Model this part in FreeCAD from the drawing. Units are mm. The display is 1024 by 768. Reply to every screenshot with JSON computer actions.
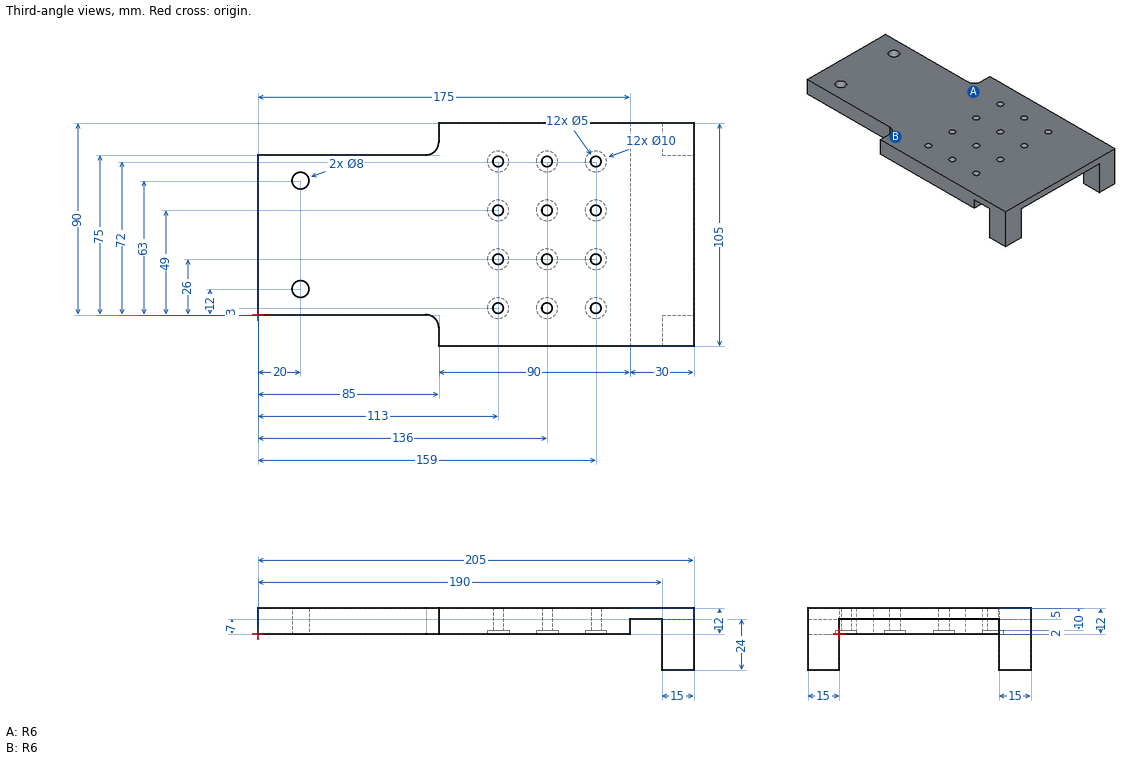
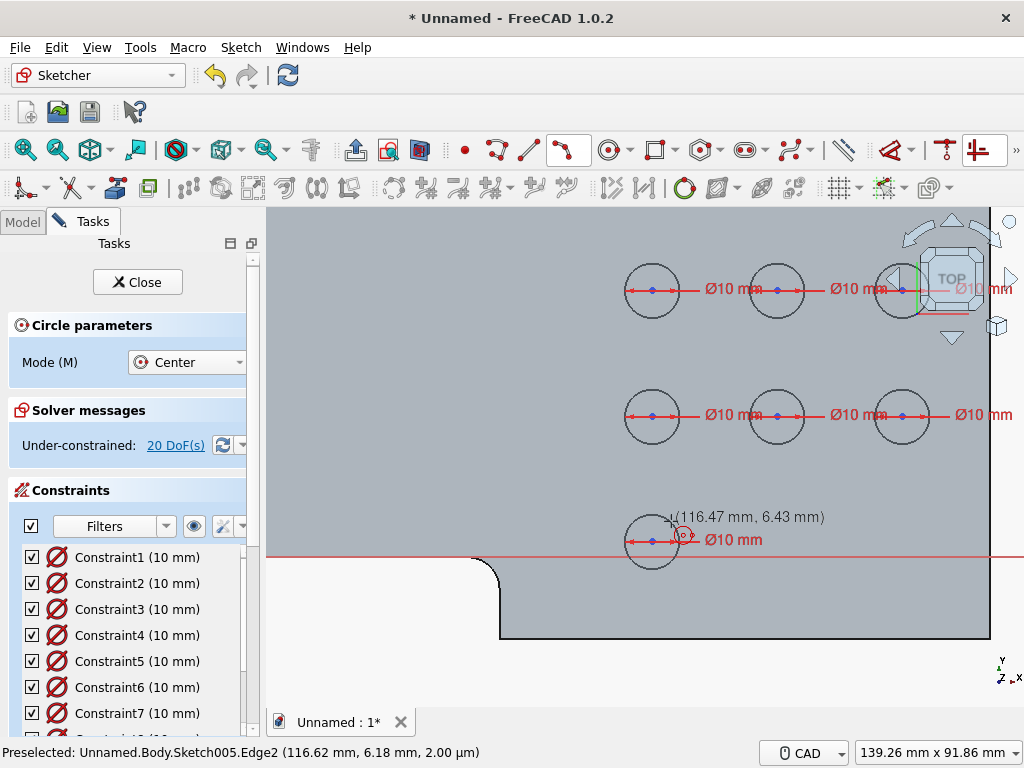
{"action": "left_click", "coordinate": [777, 541]}
{"action": "mouse_move", "coordinate": [797, 521]}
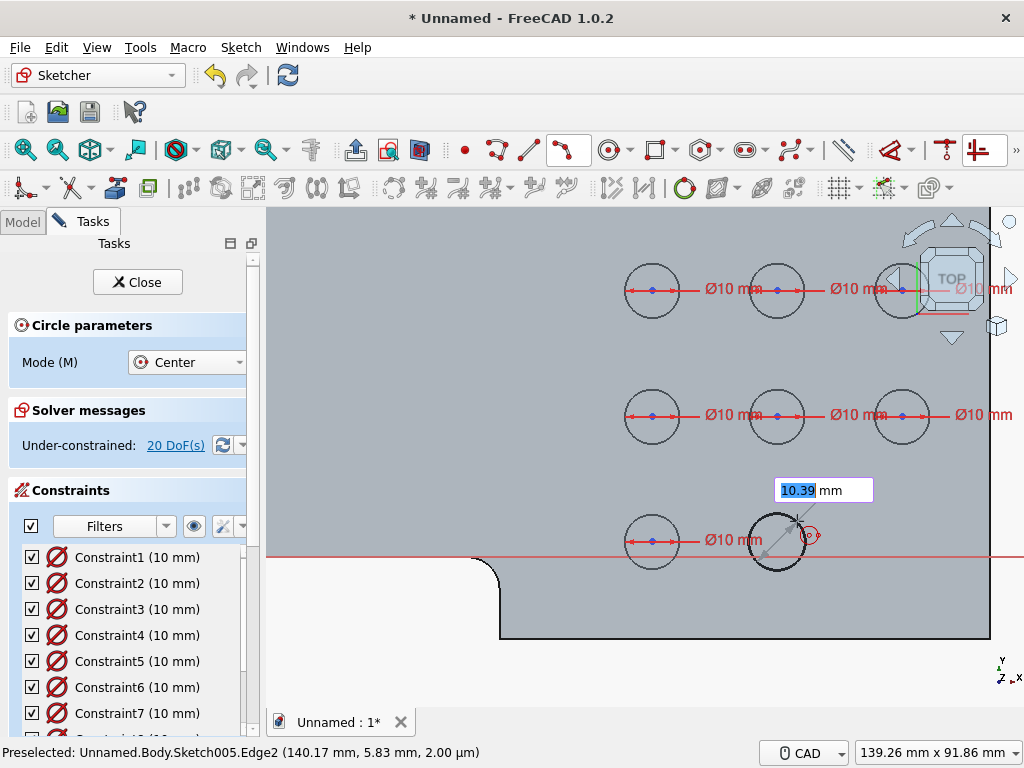
{"action": "type", "text": "10"}
{"action": "key", "text": "Return"}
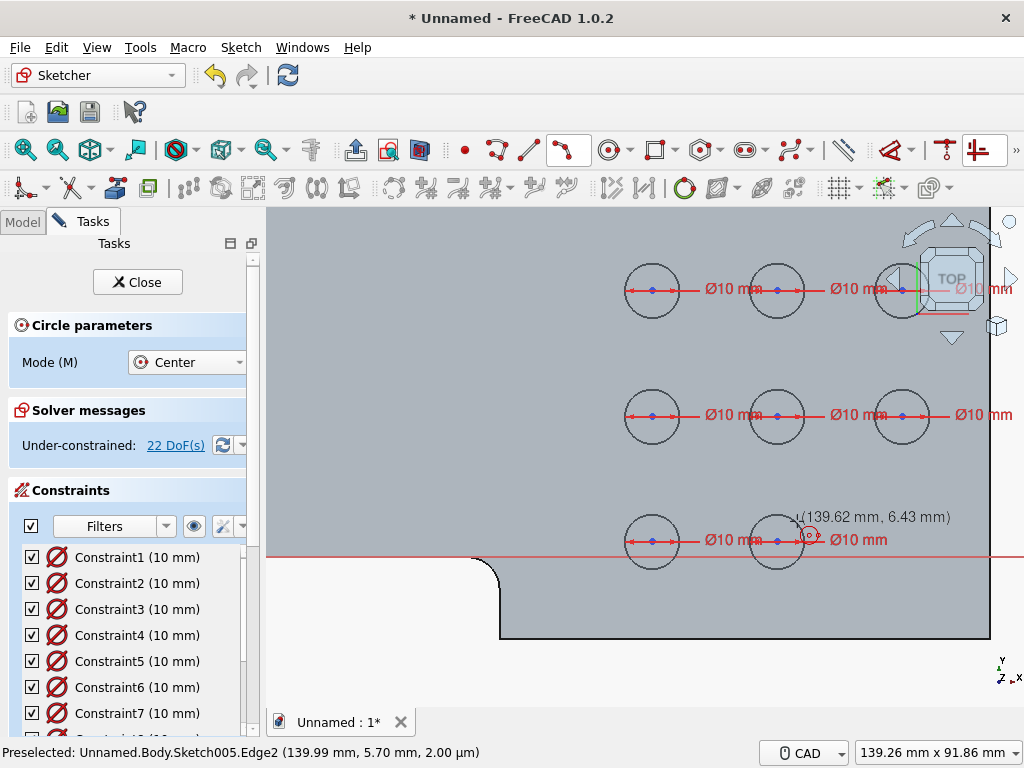
{"action": "scroll", "coordinate": [652, 542], "scroll_direction": "down", "scroll_amount": 4}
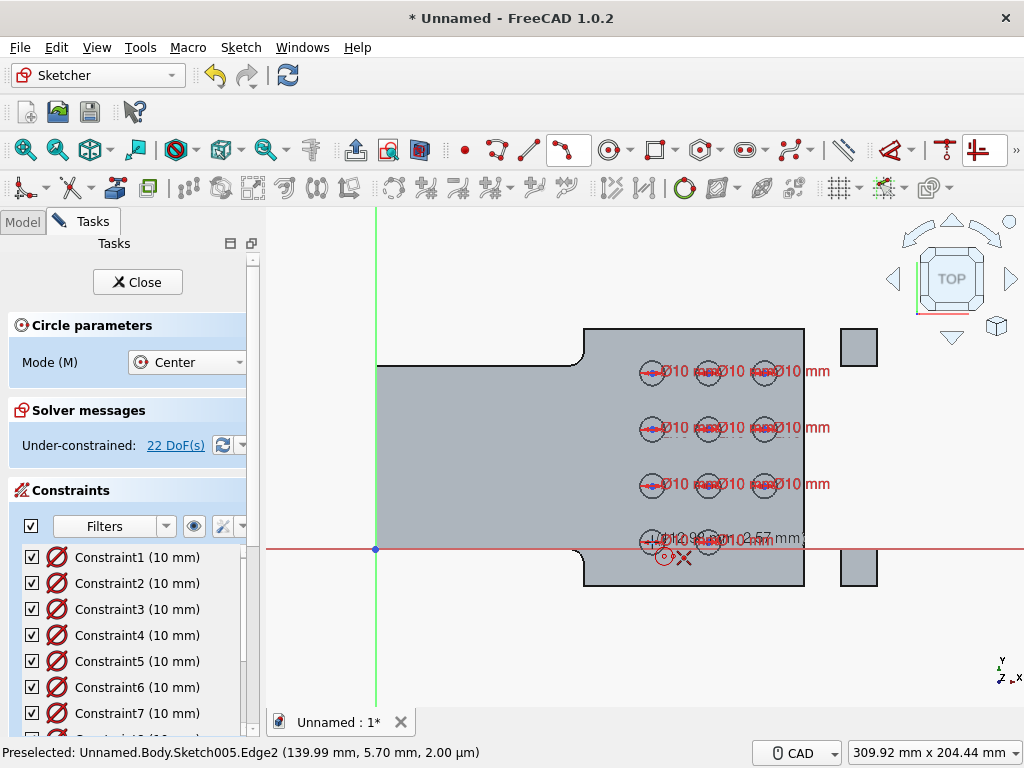
{"action": "scroll", "coordinate": [765, 542], "scroll_direction": "up", "scroll_amount": 4}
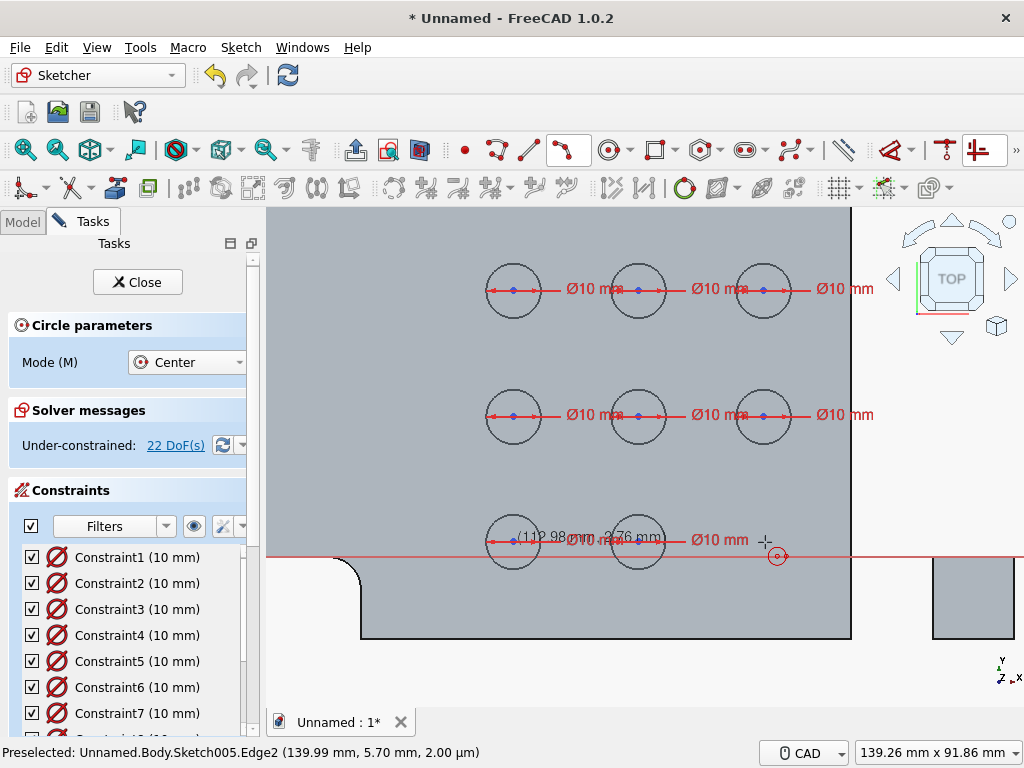
{"action": "left_click", "coordinate": [764, 541]}
{"action": "mouse_move", "coordinate": [783, 521]}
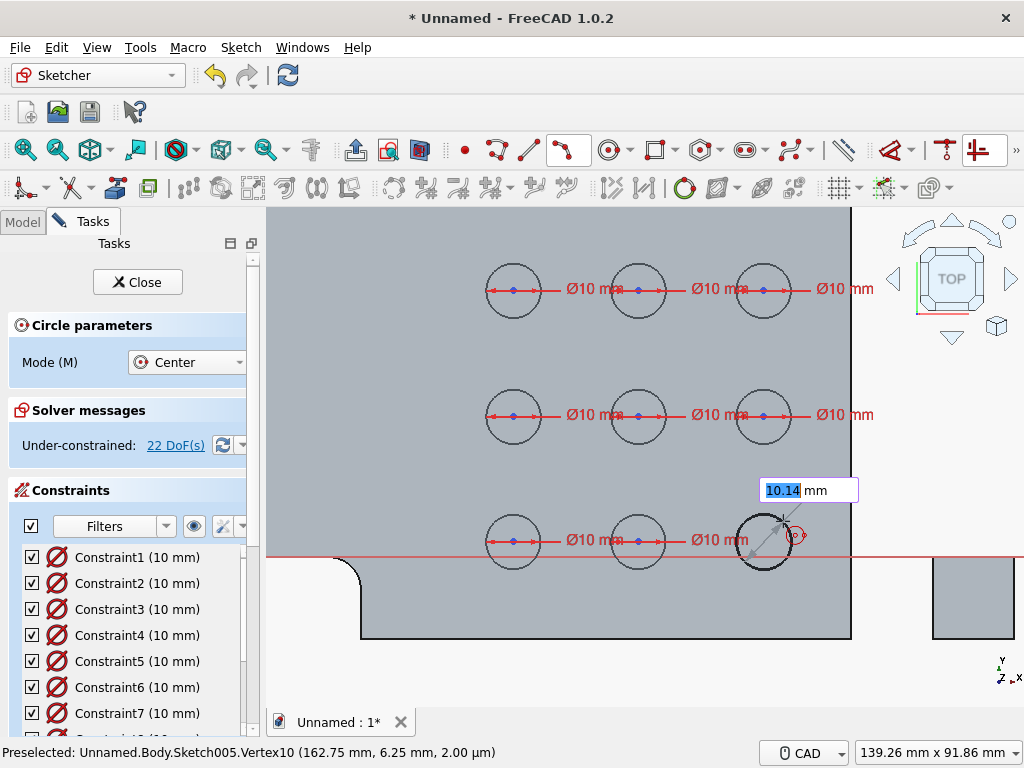
{"action": "type", "text": "10"}
{"action": "key", "text": "Return"}
{"action": "key", "text": "Escape"}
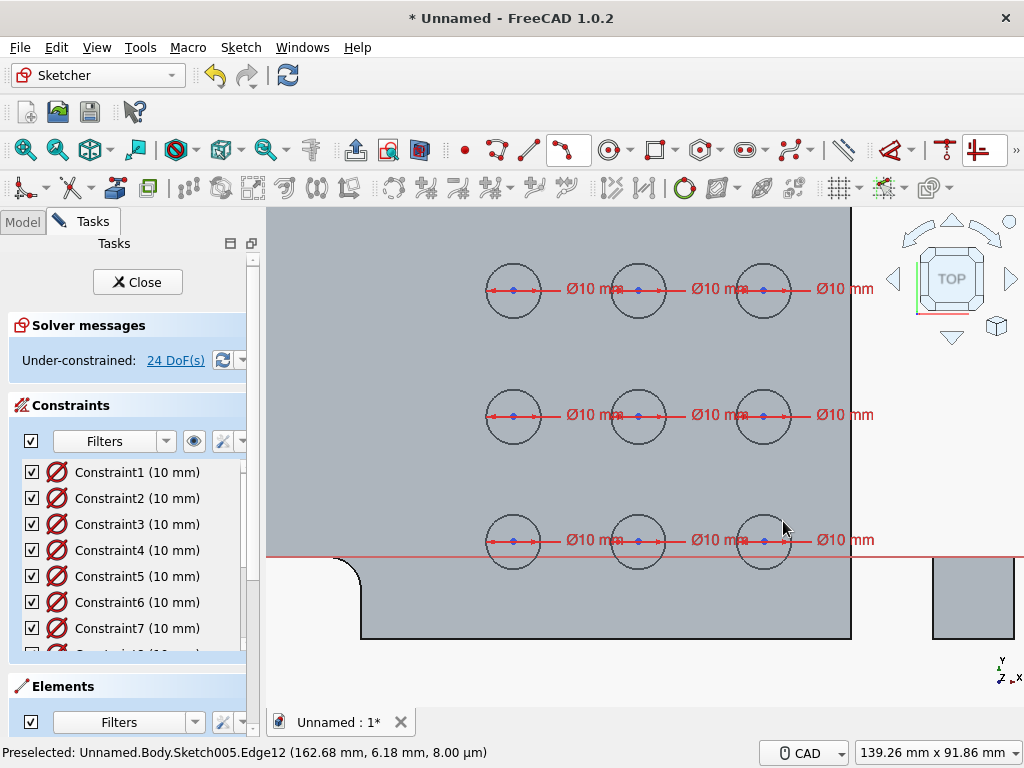
{"action": "scroll", "coordinate": [766, 542], "scroll_direction": "down", "scroll_amount": 4}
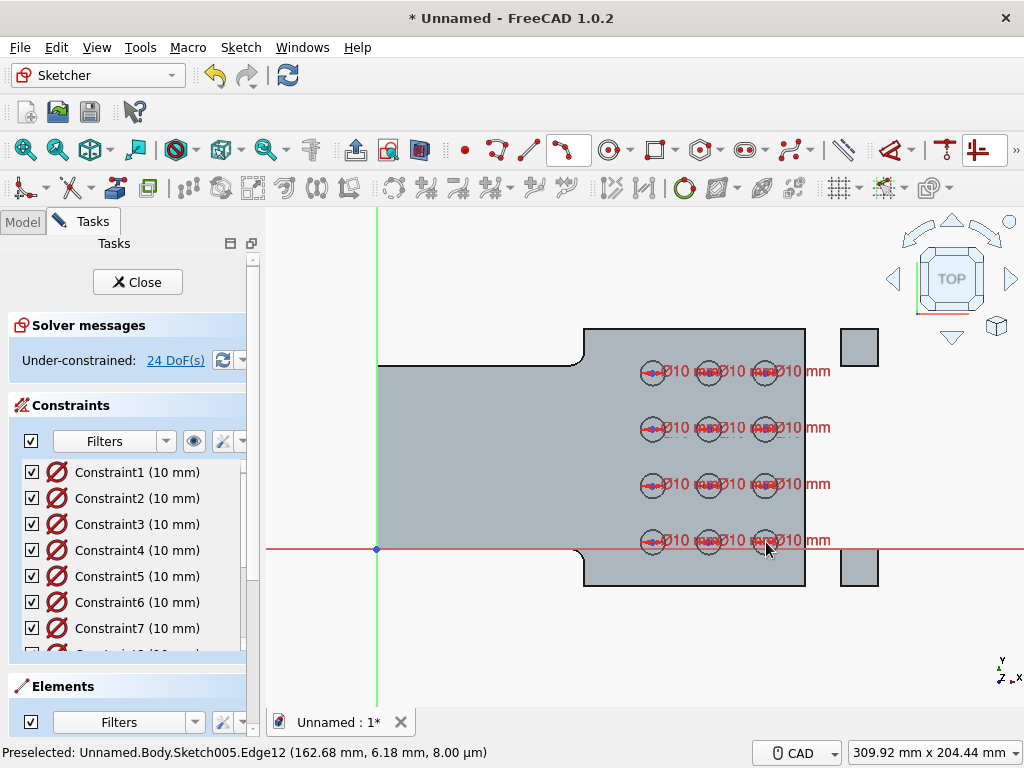
{"action": "left_click", "coordinate": [765, 373]}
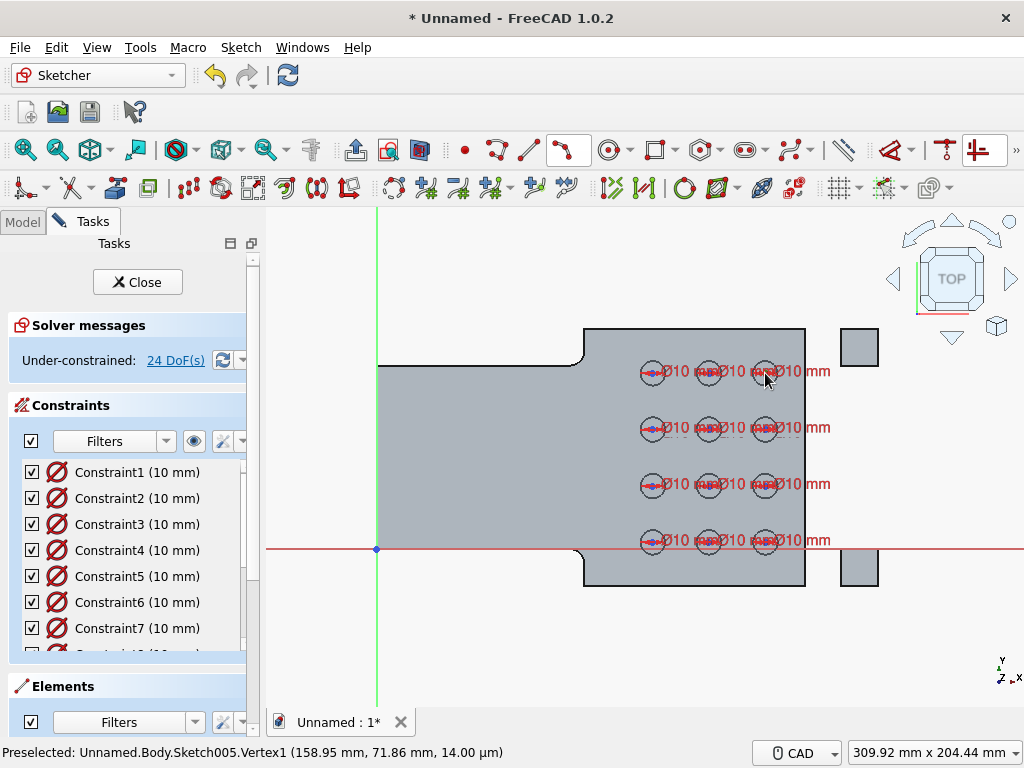
{"action": "left_click", "coordinate": [709, 373]}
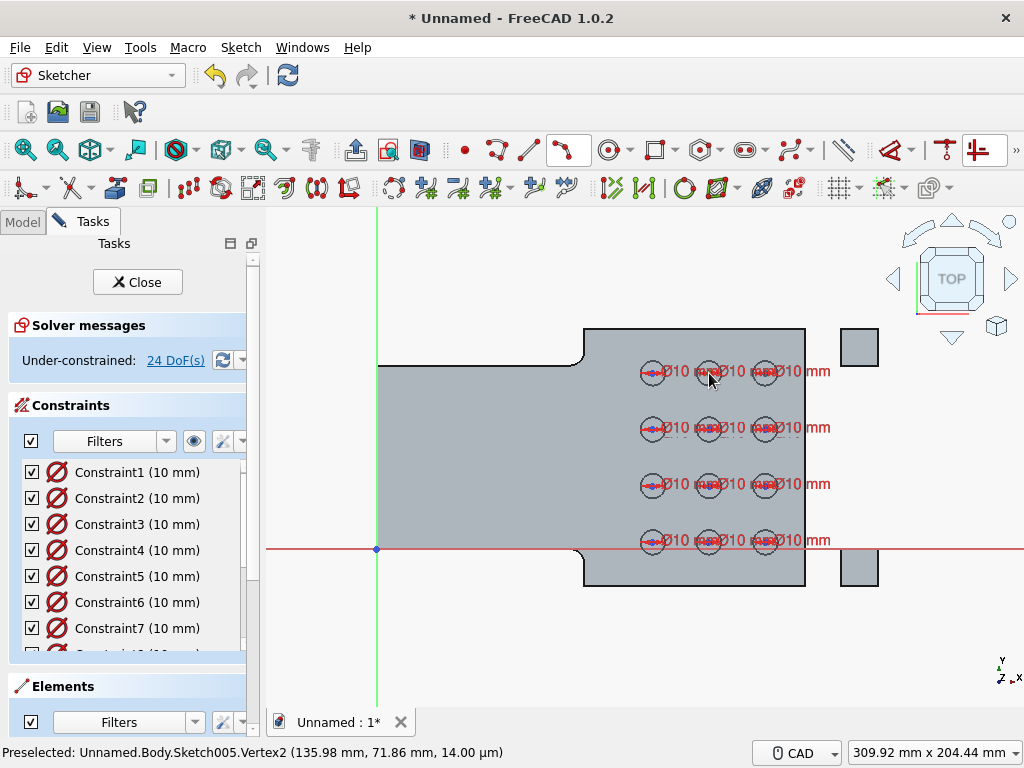
{"action": "left_click", "coordinate": [1002, 150]}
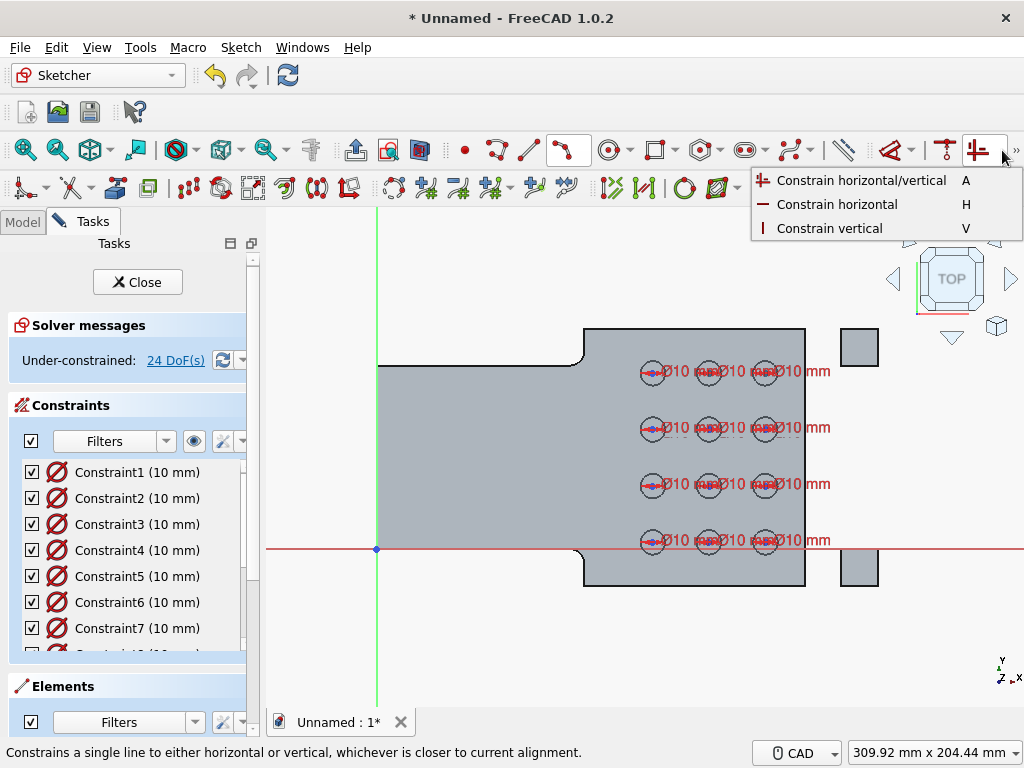
{"action": "left_click", "coordinate": [887, 204]}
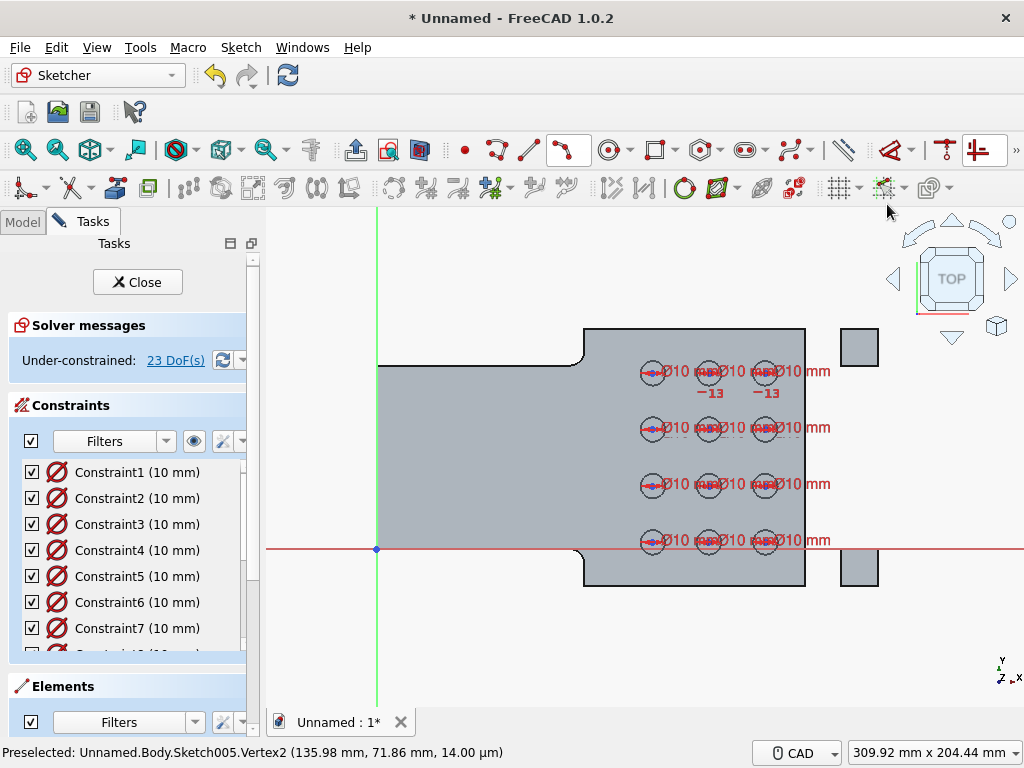
{"action": "left_click", "coordinate": [709, 373]}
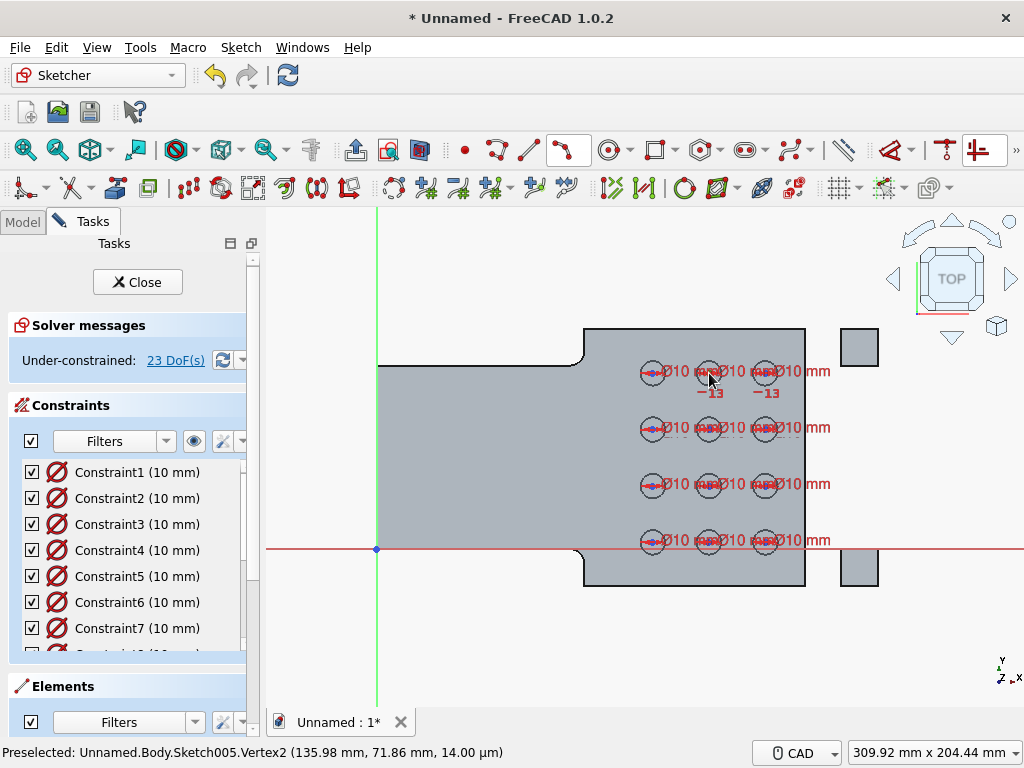
{"action": "left_click", "coordinate": [653, 373]}